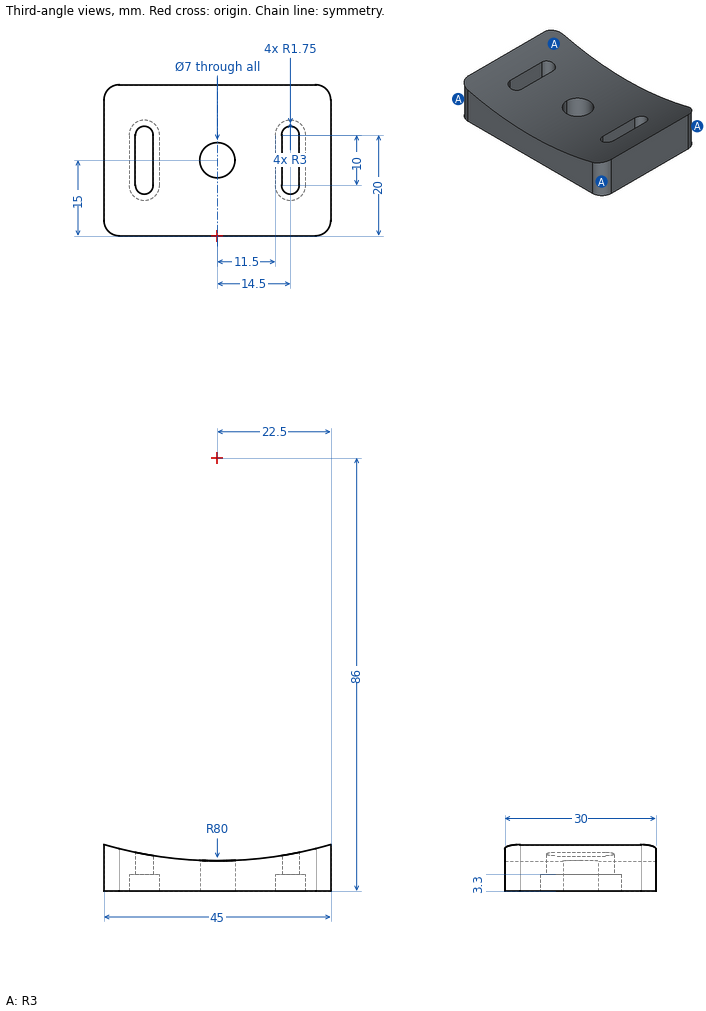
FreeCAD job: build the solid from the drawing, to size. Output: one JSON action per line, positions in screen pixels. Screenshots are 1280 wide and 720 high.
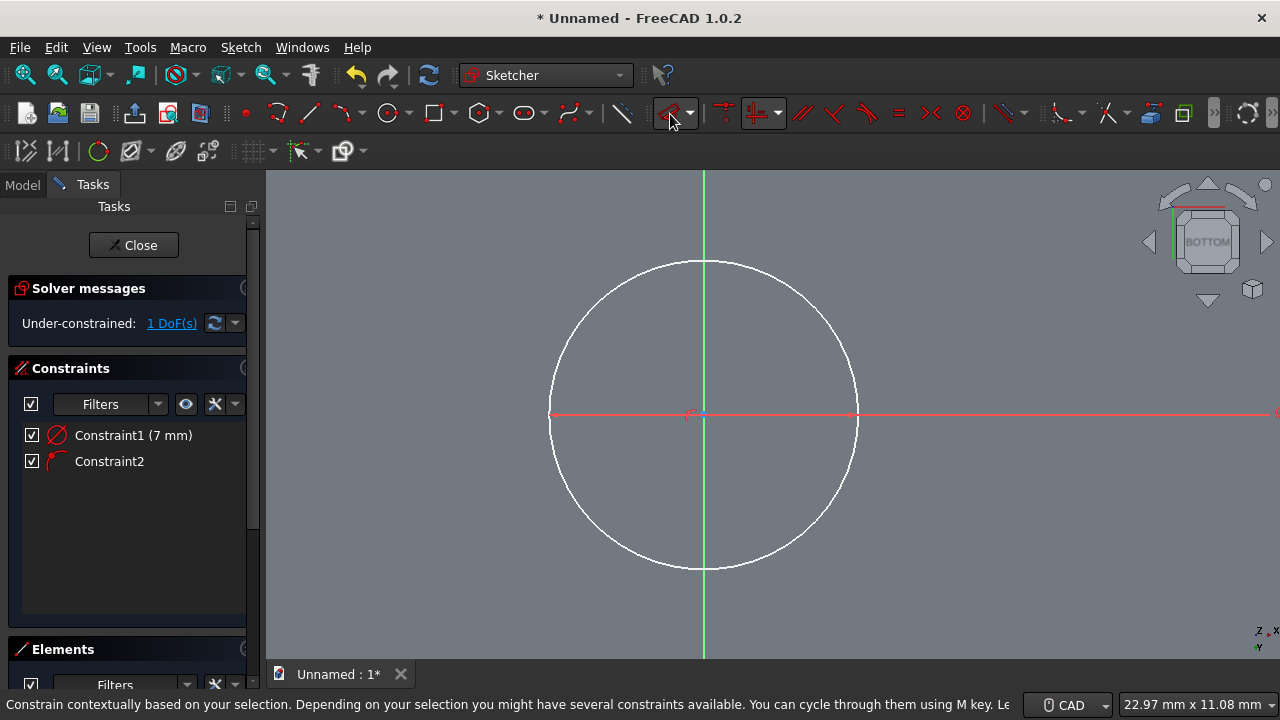
{"action": "left_click", "coordinate": [704, 415]}
{"action": "left_click", "coordinate": [738, 306]}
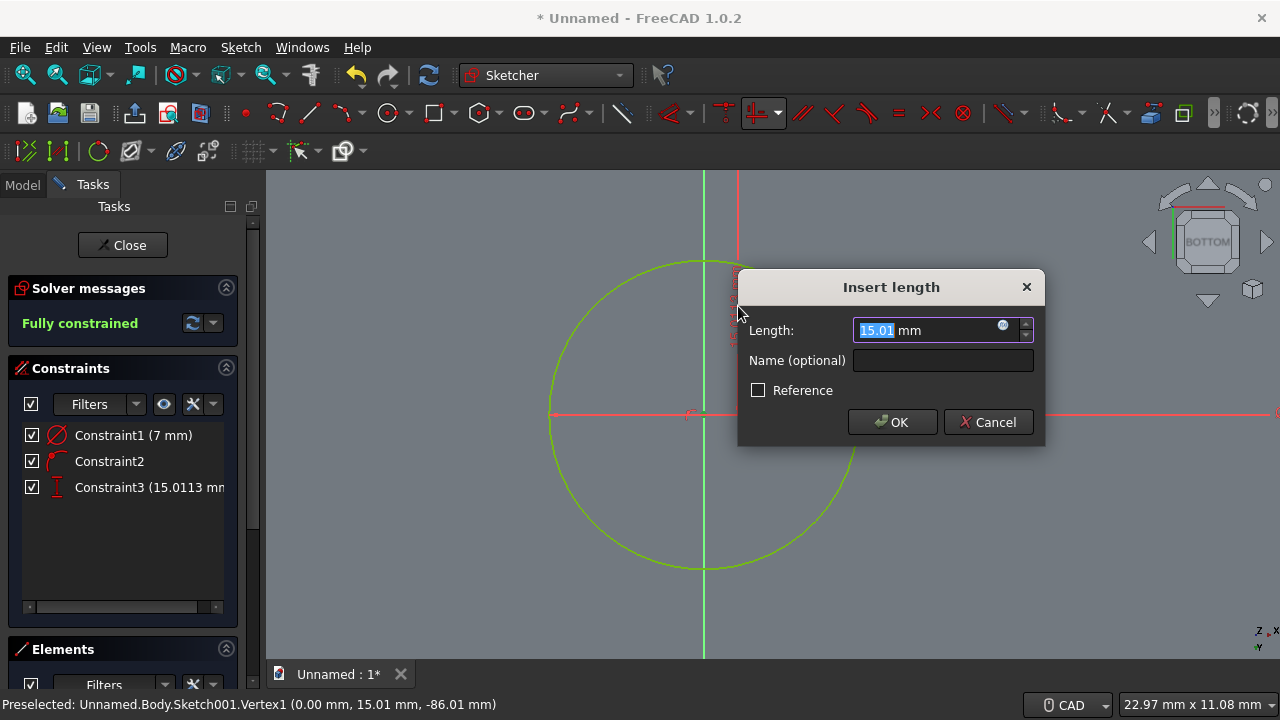
{"action": "type", "text": "15"}
{"action": "key", "text": "Return"}
{"action": "key", "text": "Escape"}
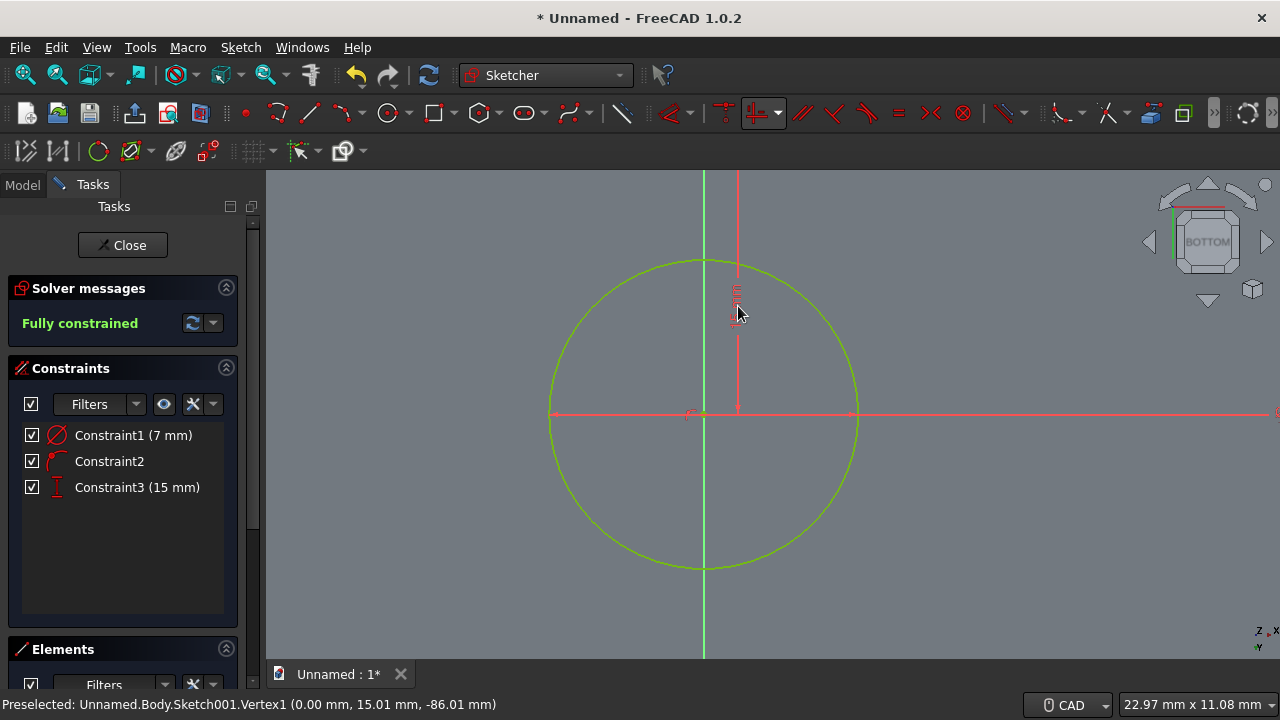
{"action": "left_click", "coordinate": [123, 245]}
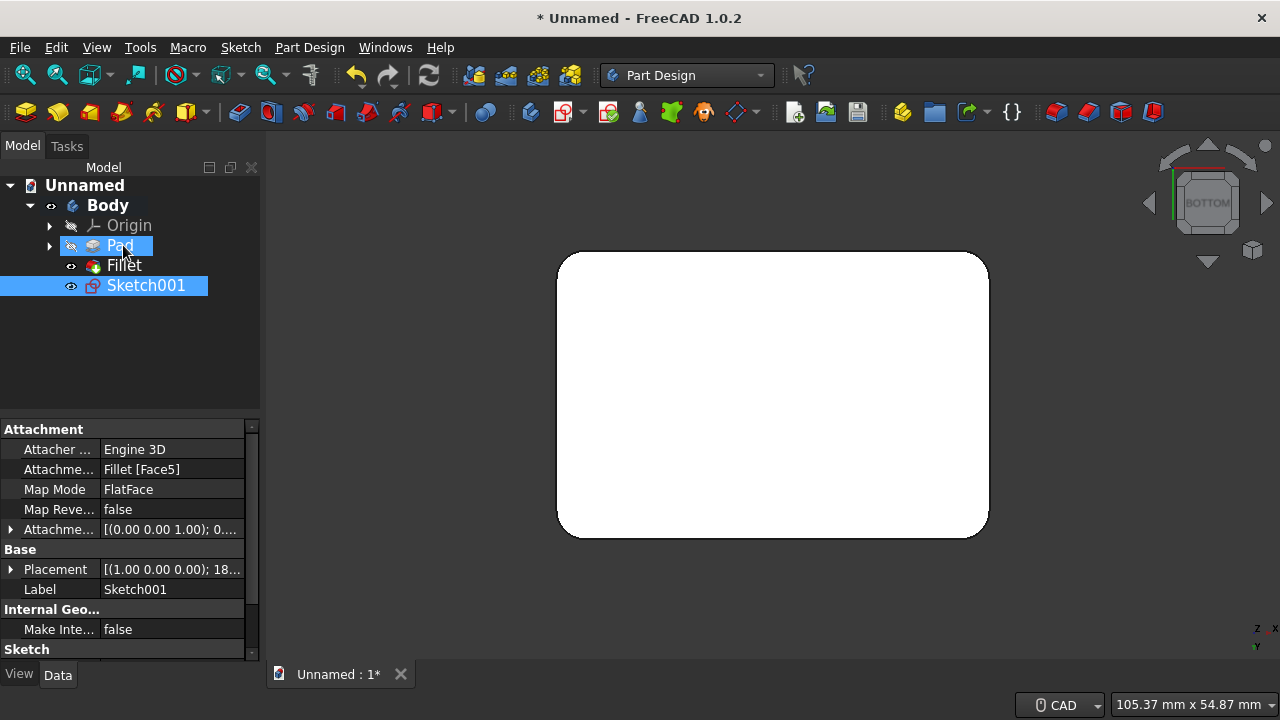
{"action": "left_click", "coordinate": [272, 112]}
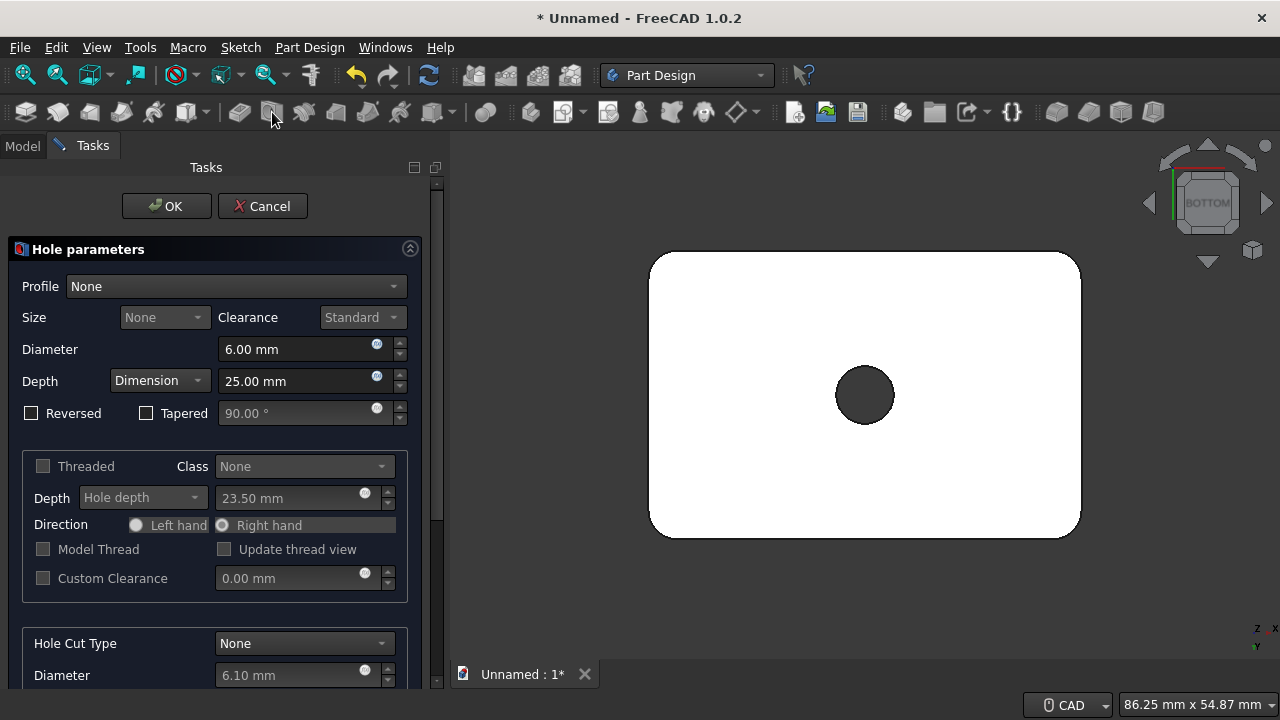
{"action": "triple_click", "coordinate": [305, 349]}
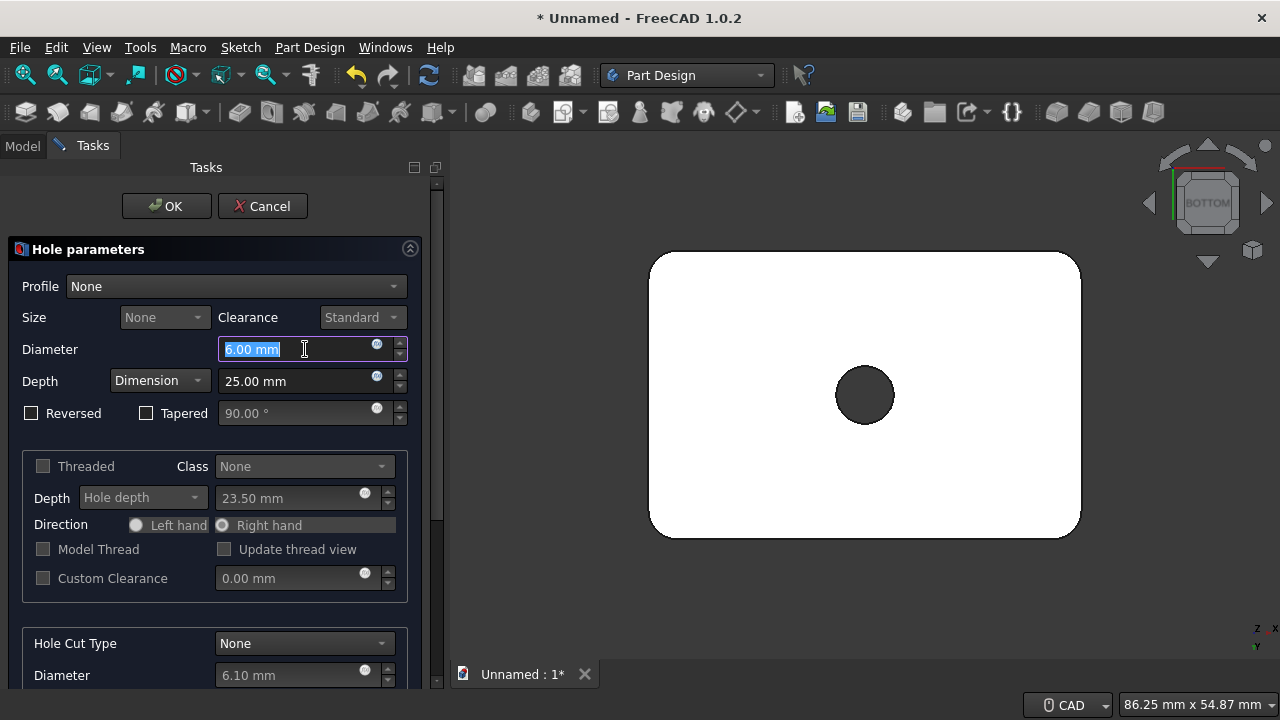
{"action": "type", "text": "7"}
{"action": "key", "text": "Tab"}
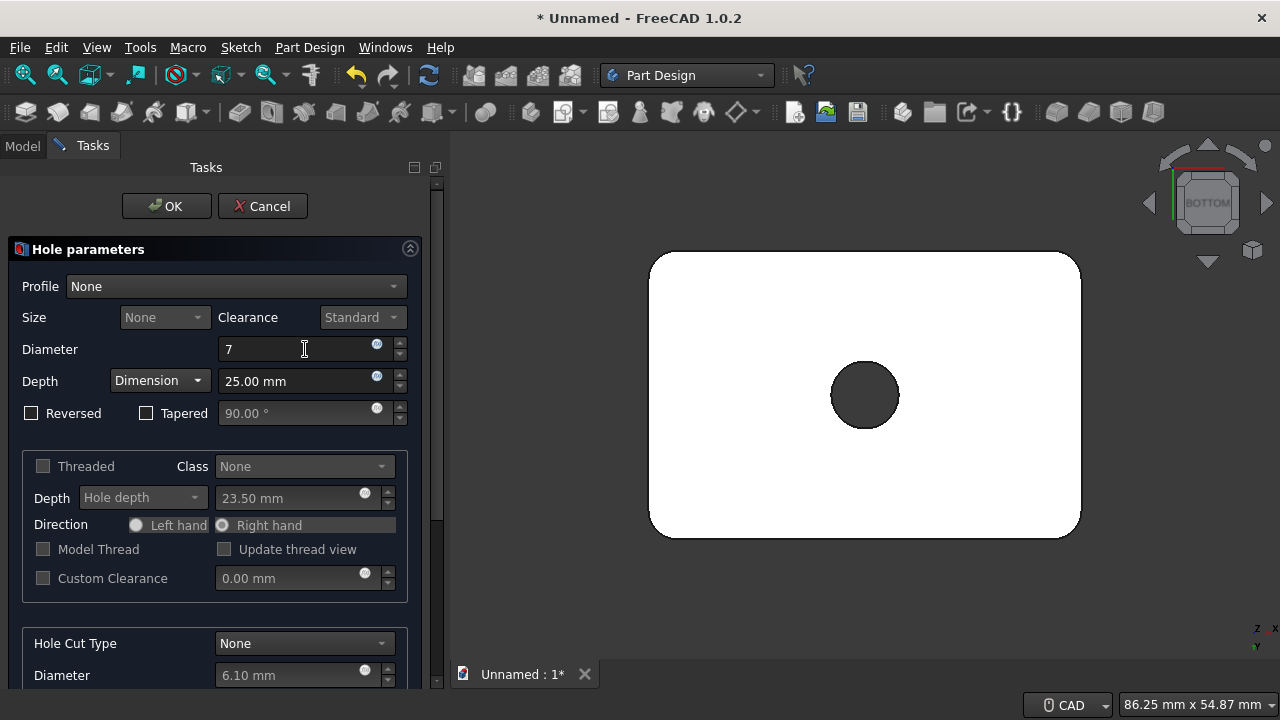
{"action": "left_click", "coordinate": [161, 380]}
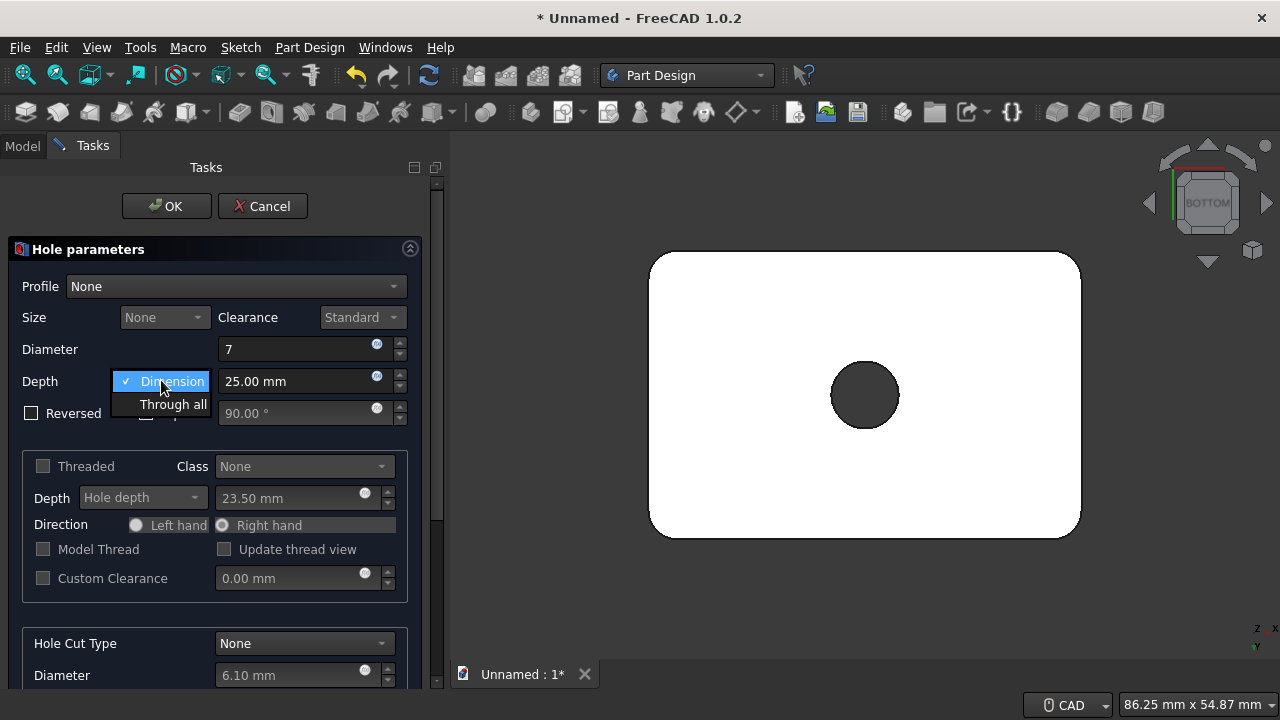
{"action": "left_click", "coordinate": [160, 404]}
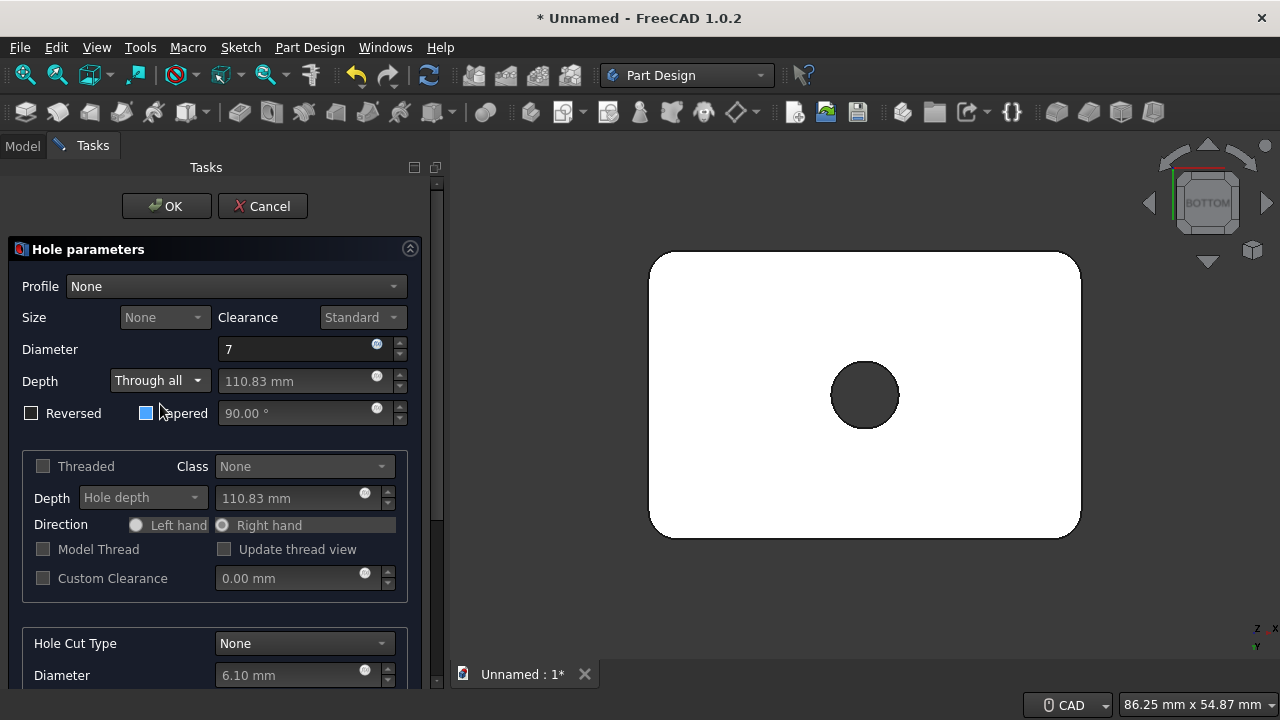
{"action": "left_click", "coordinate": [167, 206]}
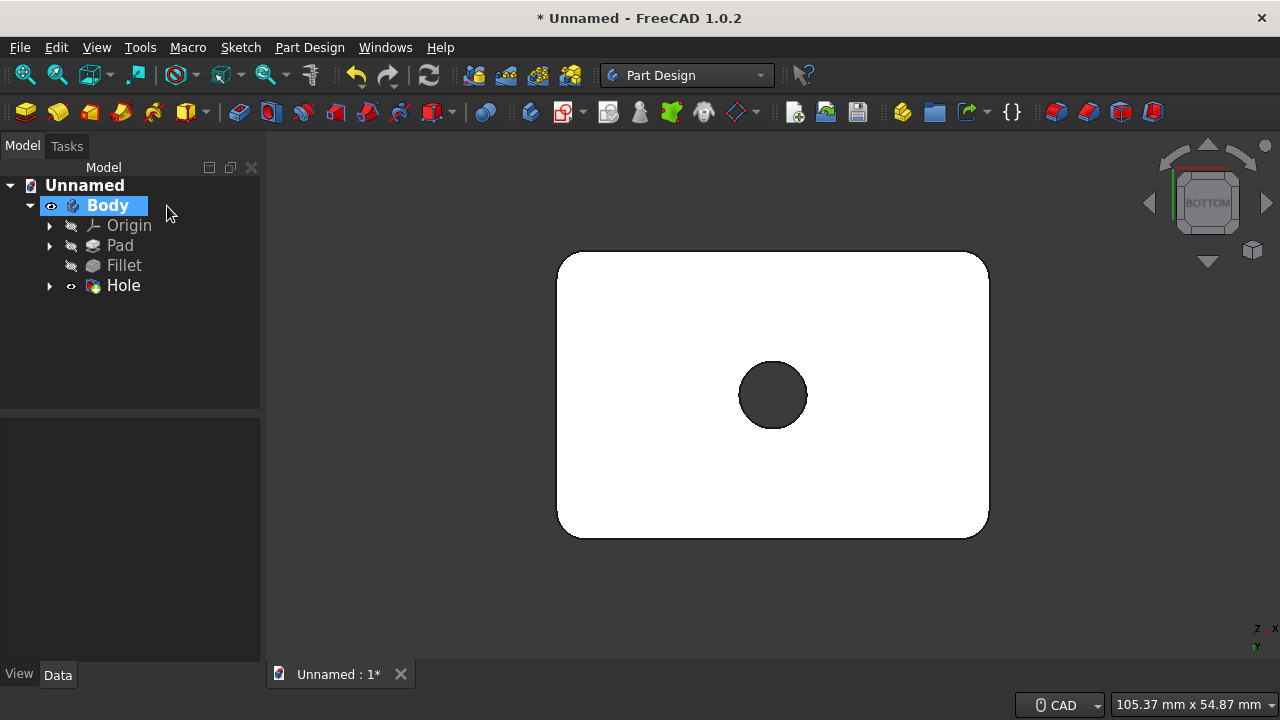
{"action": "left_click", "coordinate": [897, 435]}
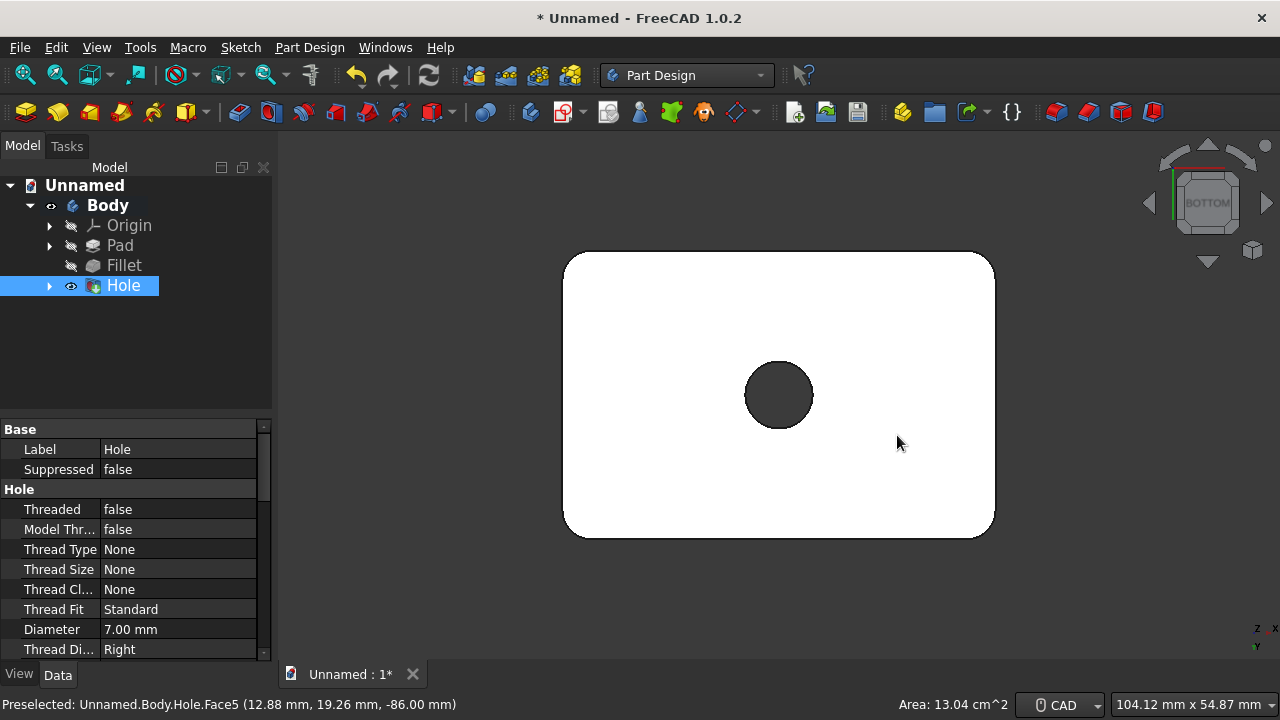
{"action": "left_click", "coordinate": [564, 112]}